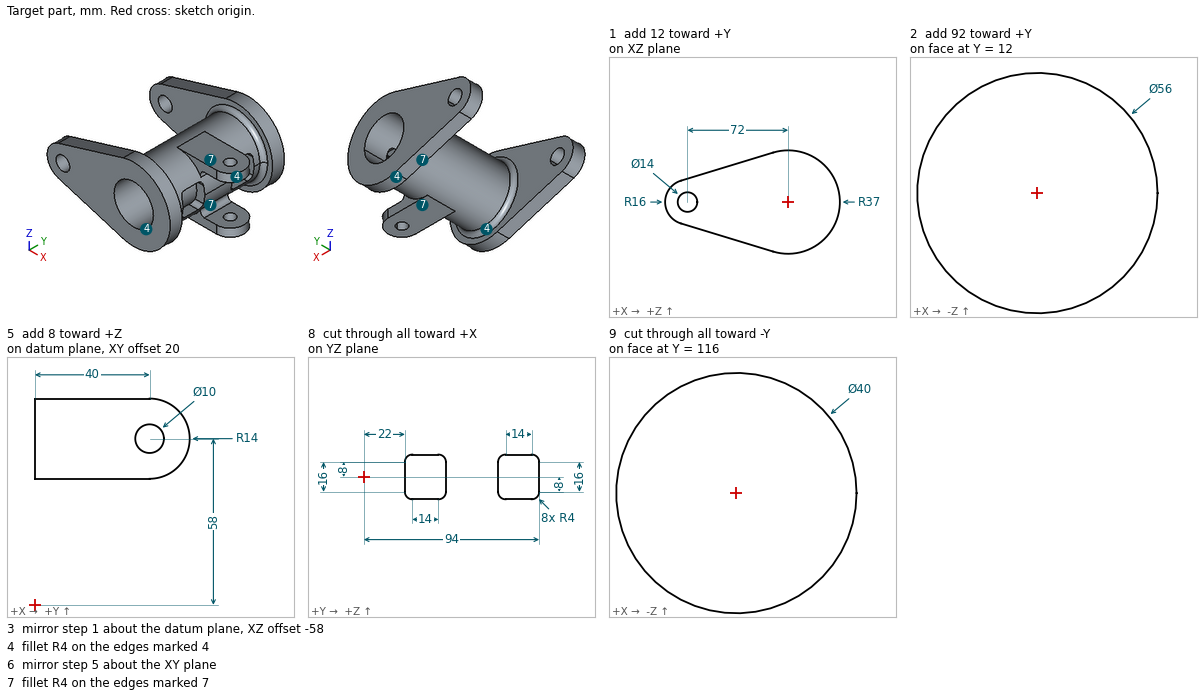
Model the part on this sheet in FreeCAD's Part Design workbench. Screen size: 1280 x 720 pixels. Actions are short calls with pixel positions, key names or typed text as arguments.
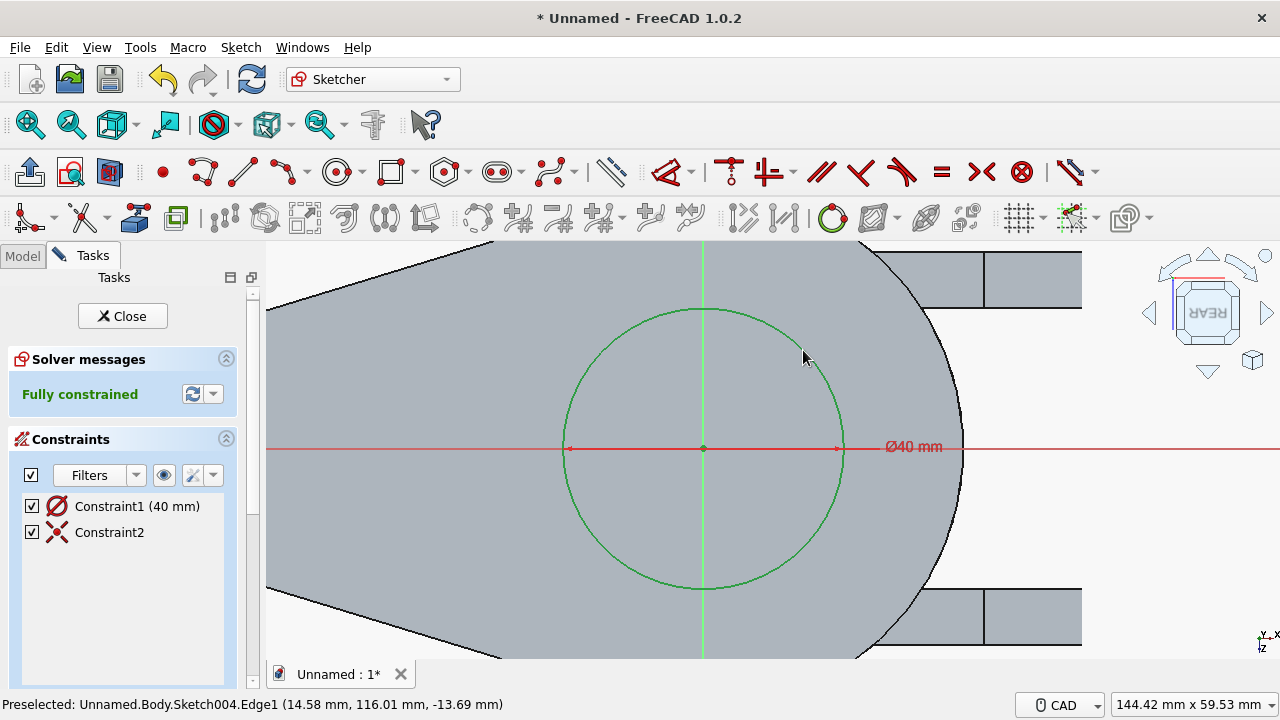
click(123, 316)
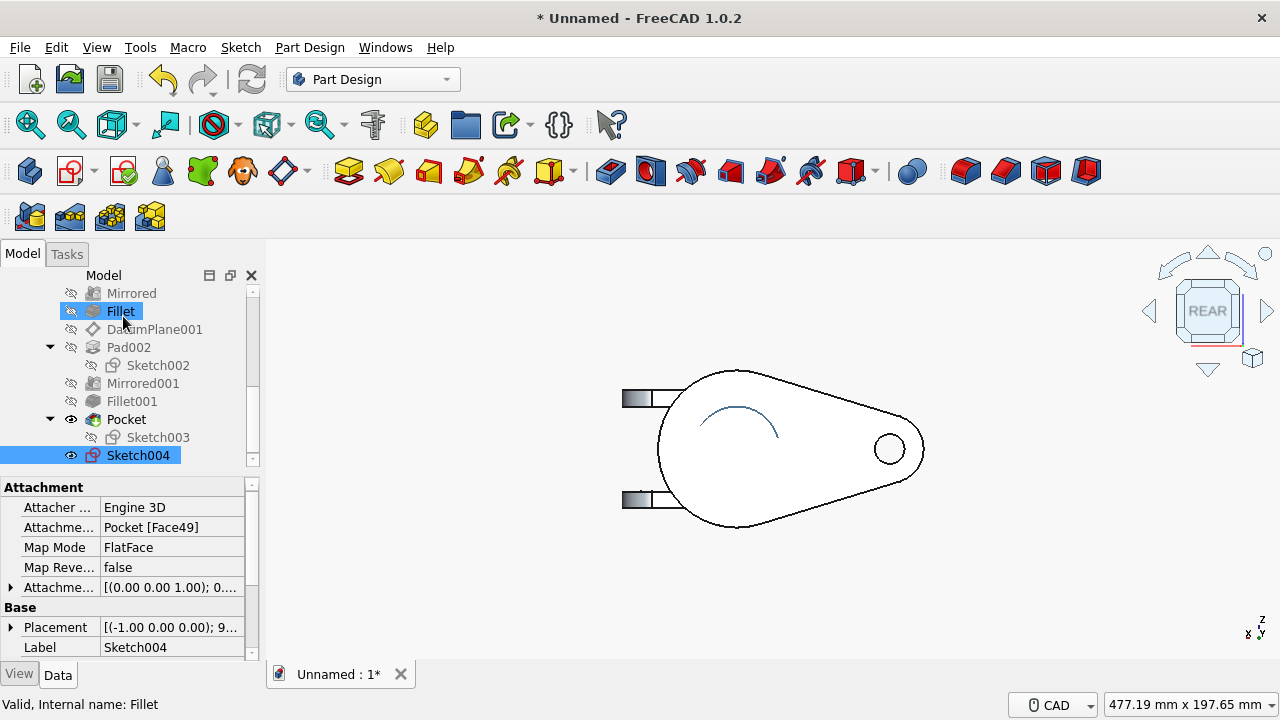
click(612, 172)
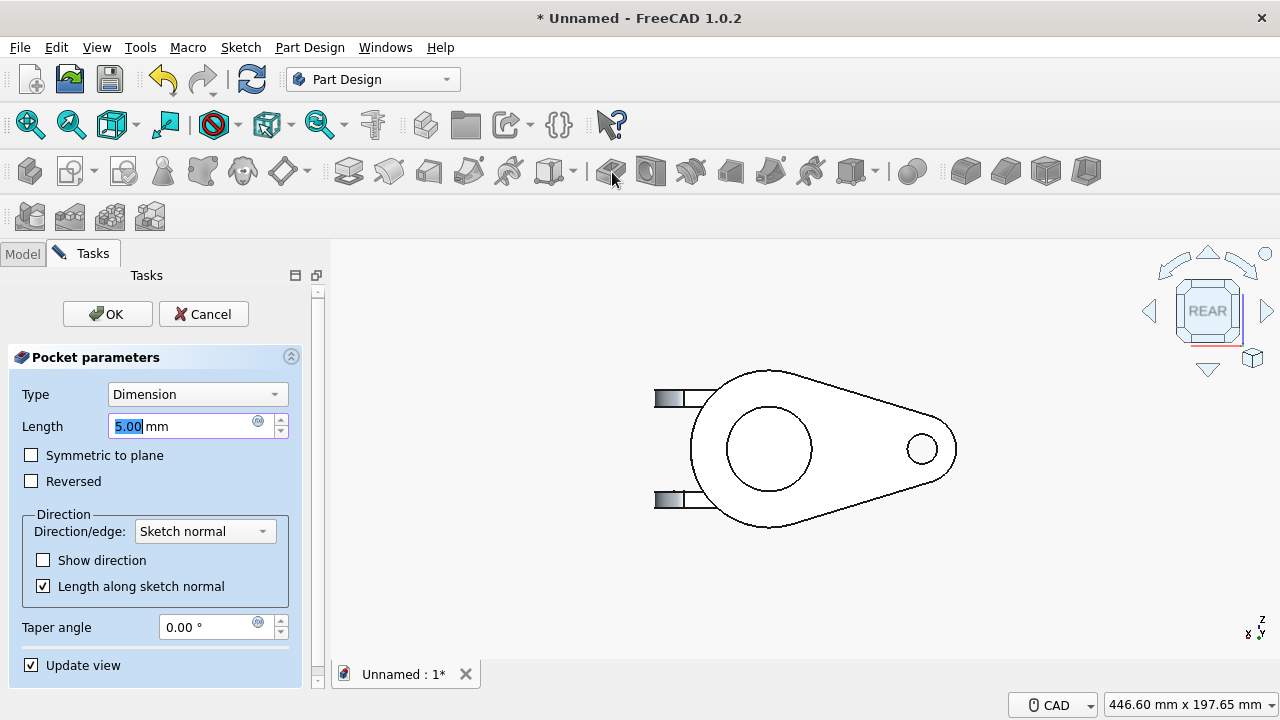
click(198, 394)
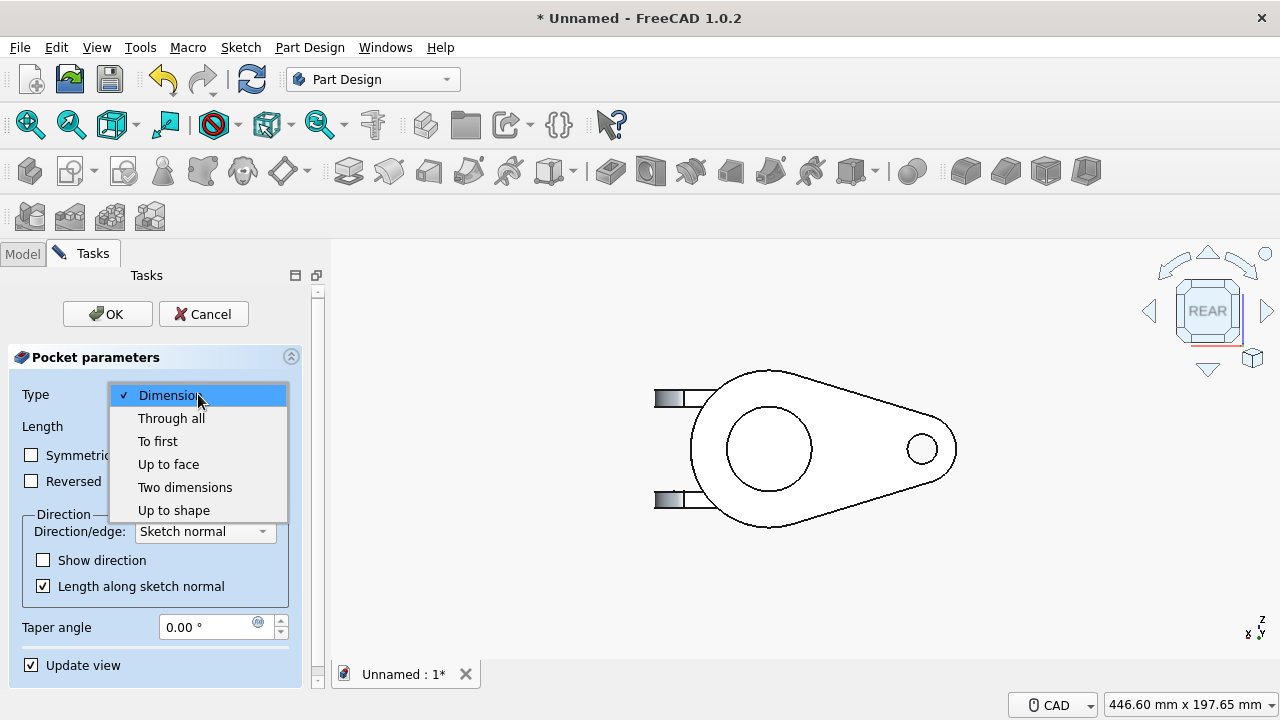
click(198, 418)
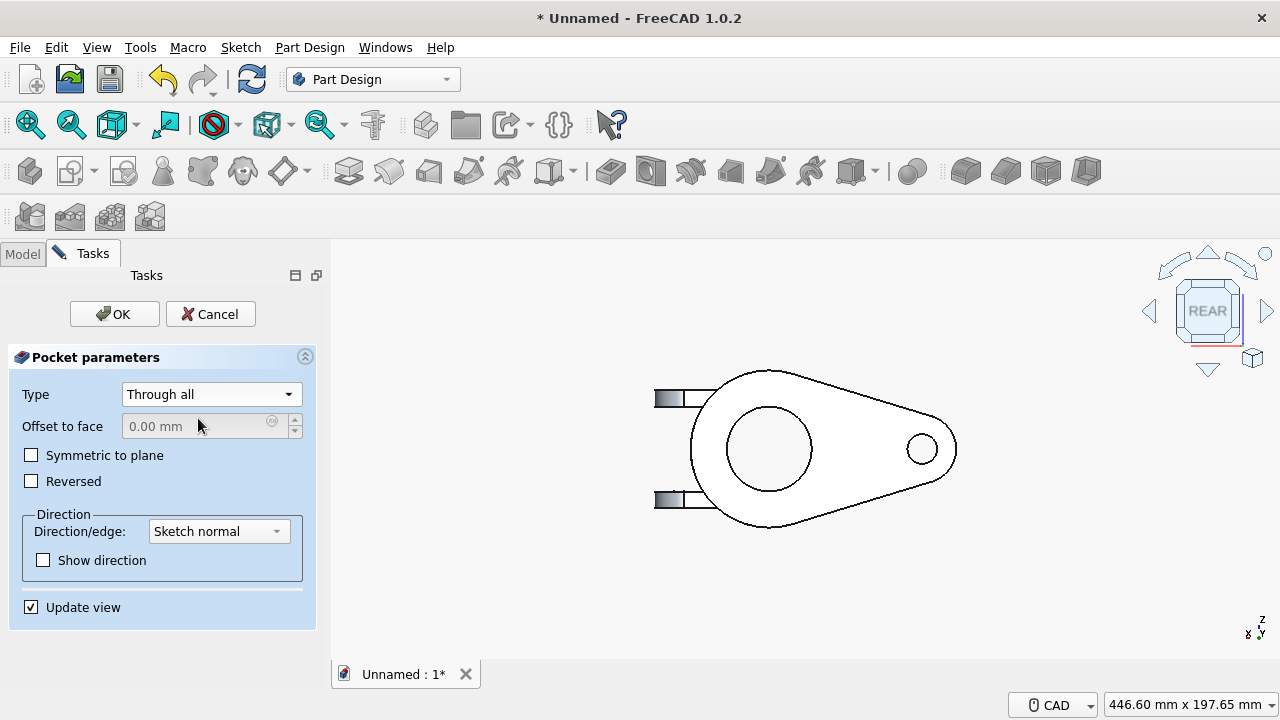
click(115, 314)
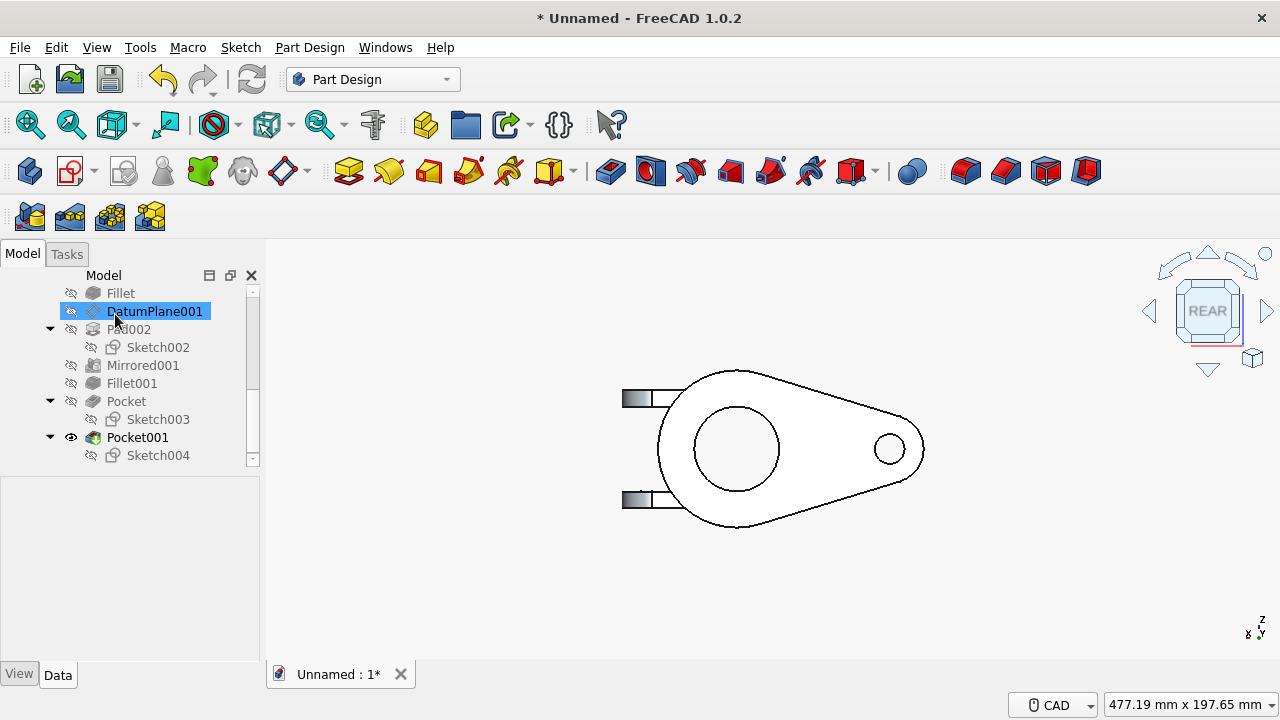
key(0)